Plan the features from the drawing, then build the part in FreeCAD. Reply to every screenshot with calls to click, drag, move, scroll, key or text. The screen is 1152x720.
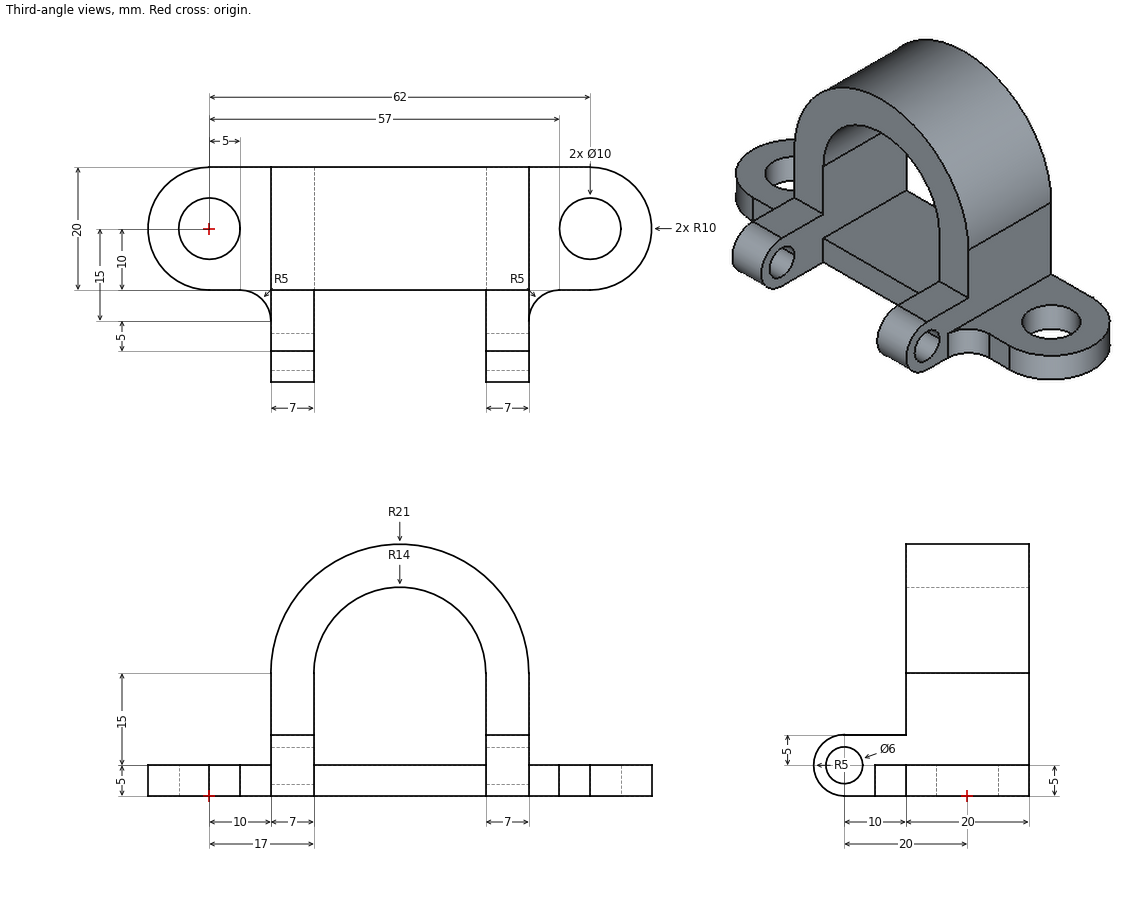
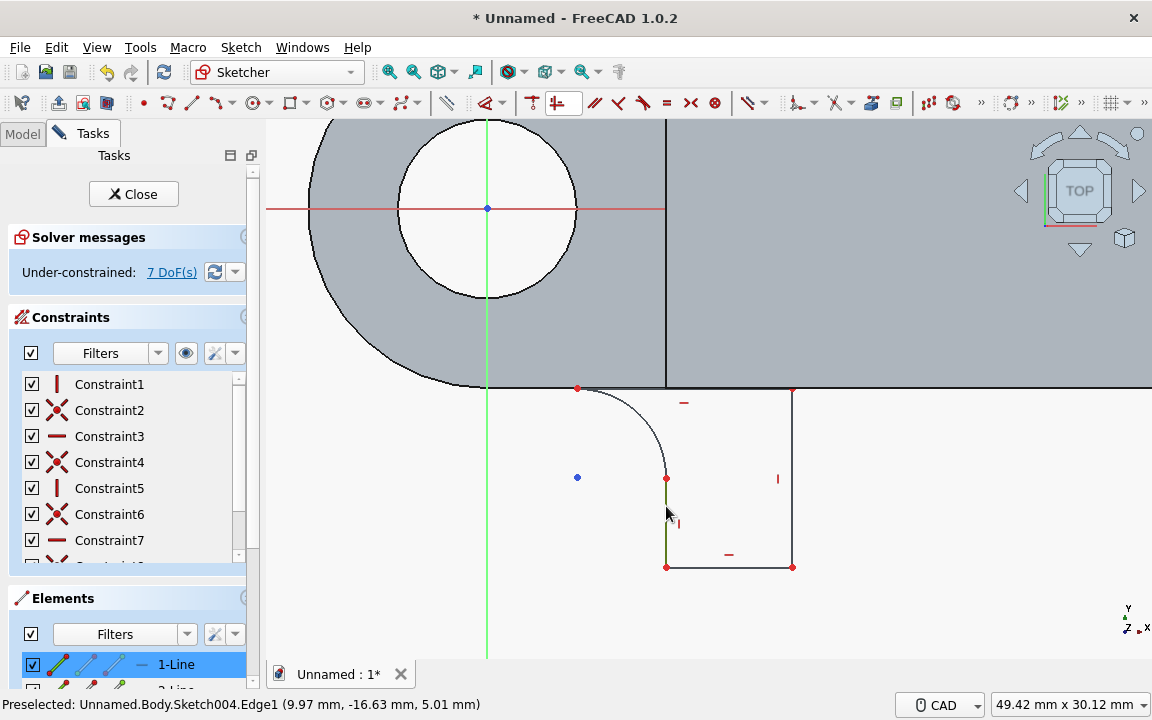
click(657, 438)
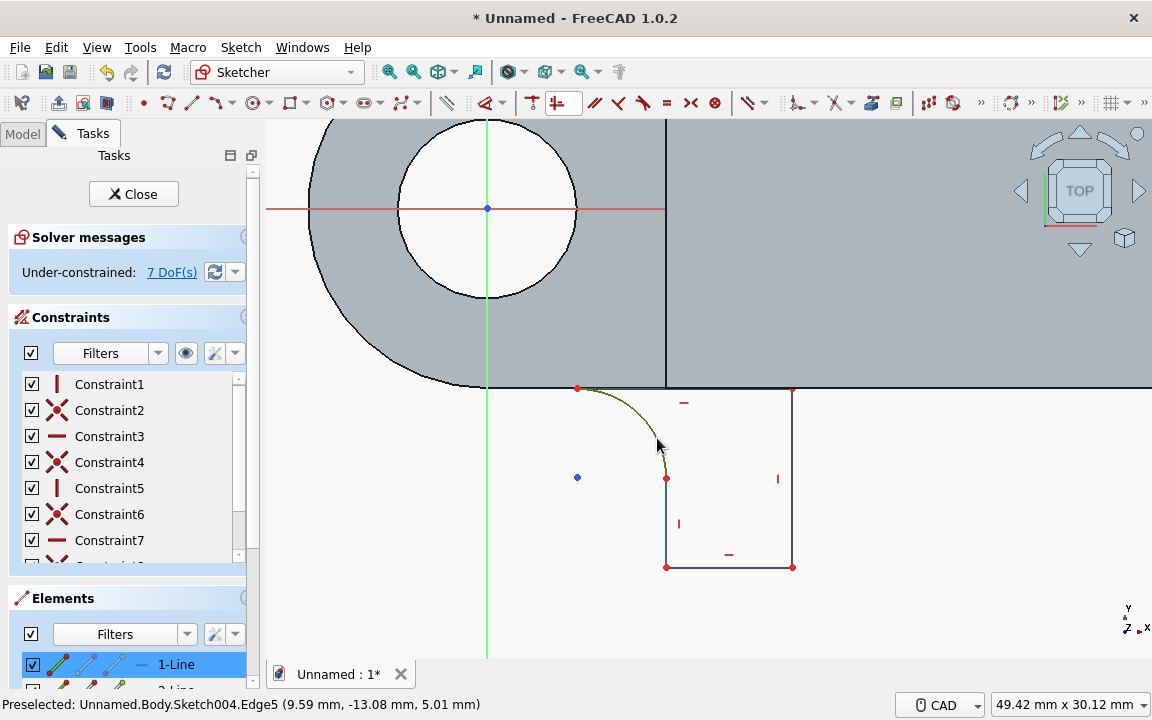
click(644, 104)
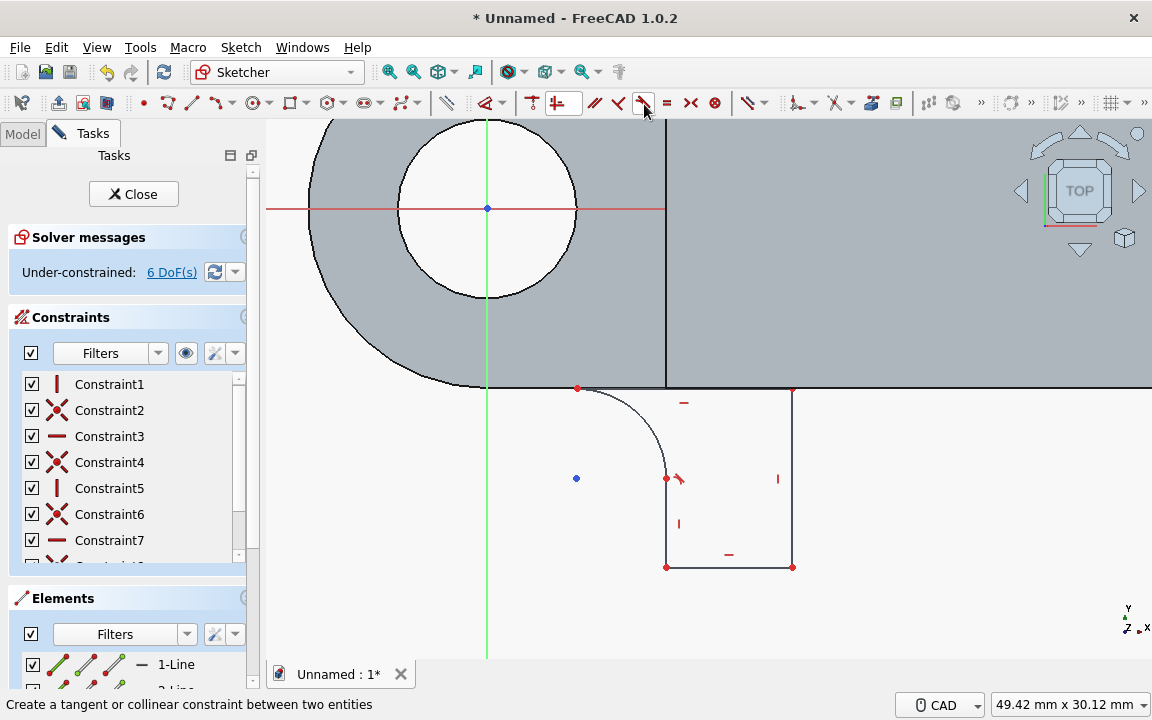
click(728, 389)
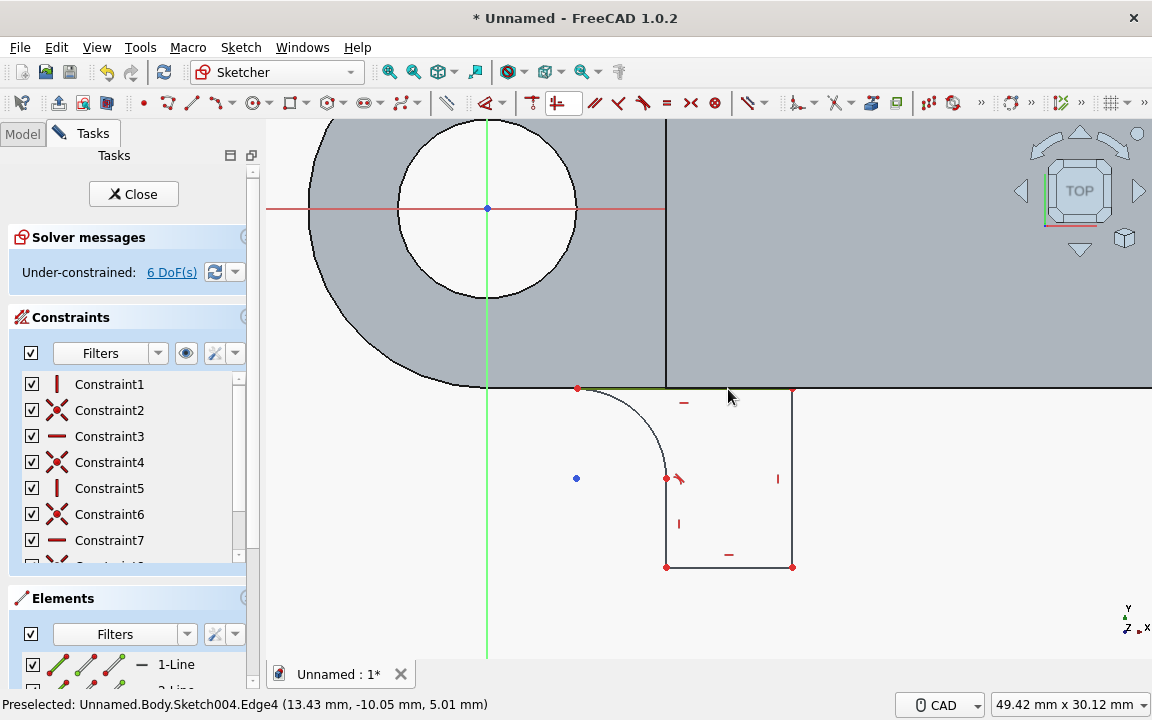
click(656, 438)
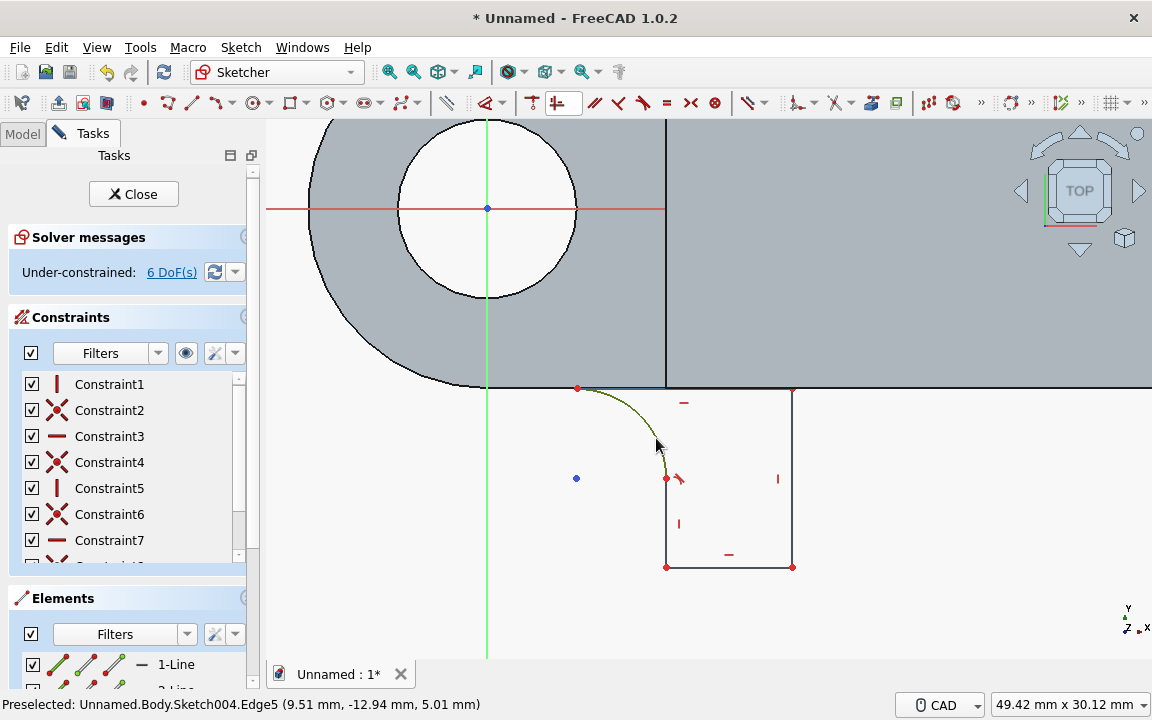
click(644, 104)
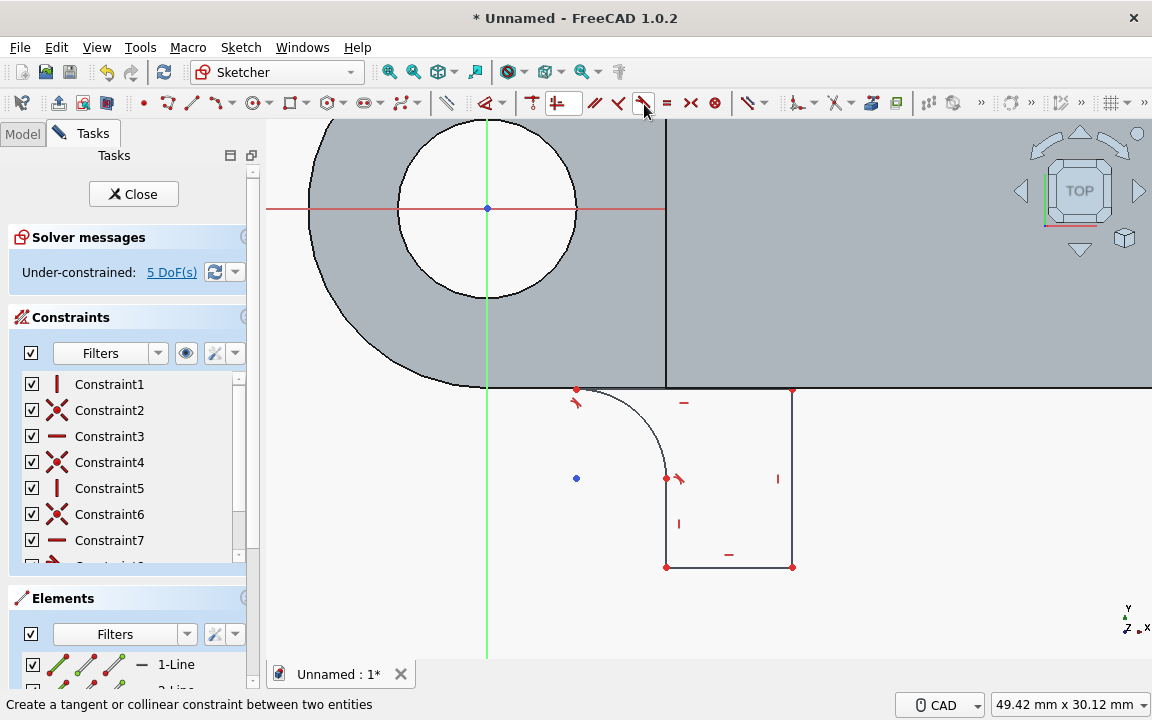
key(d)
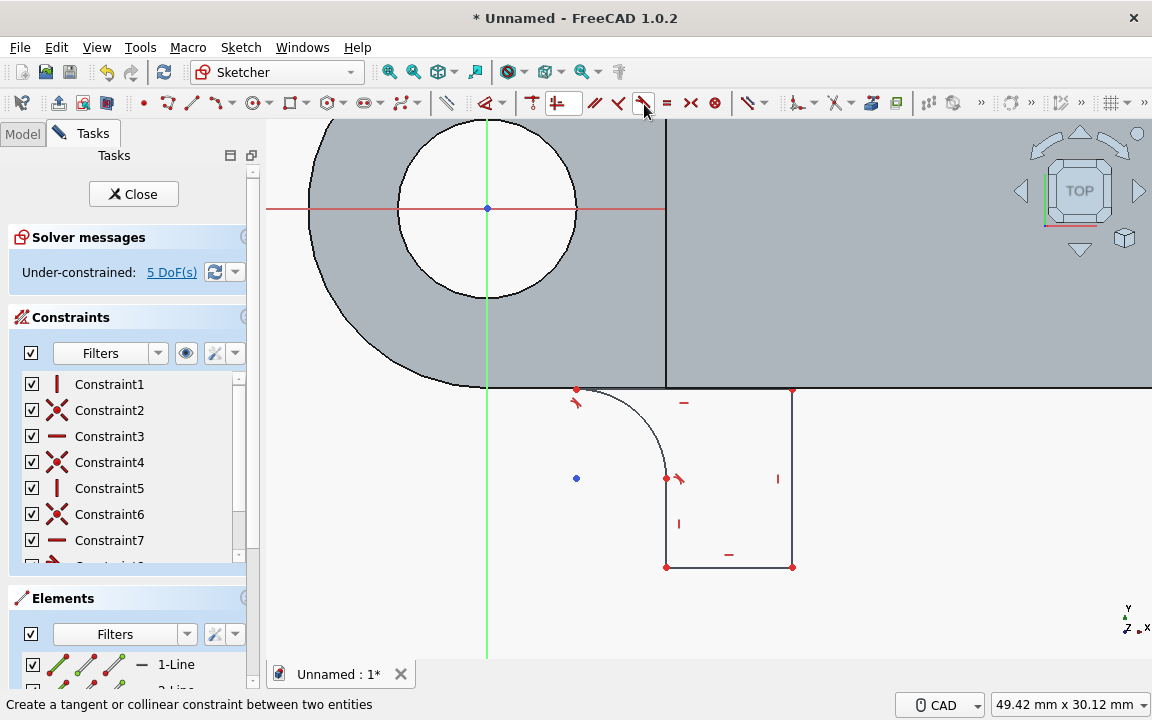
click(656, 438)
click(684, 423)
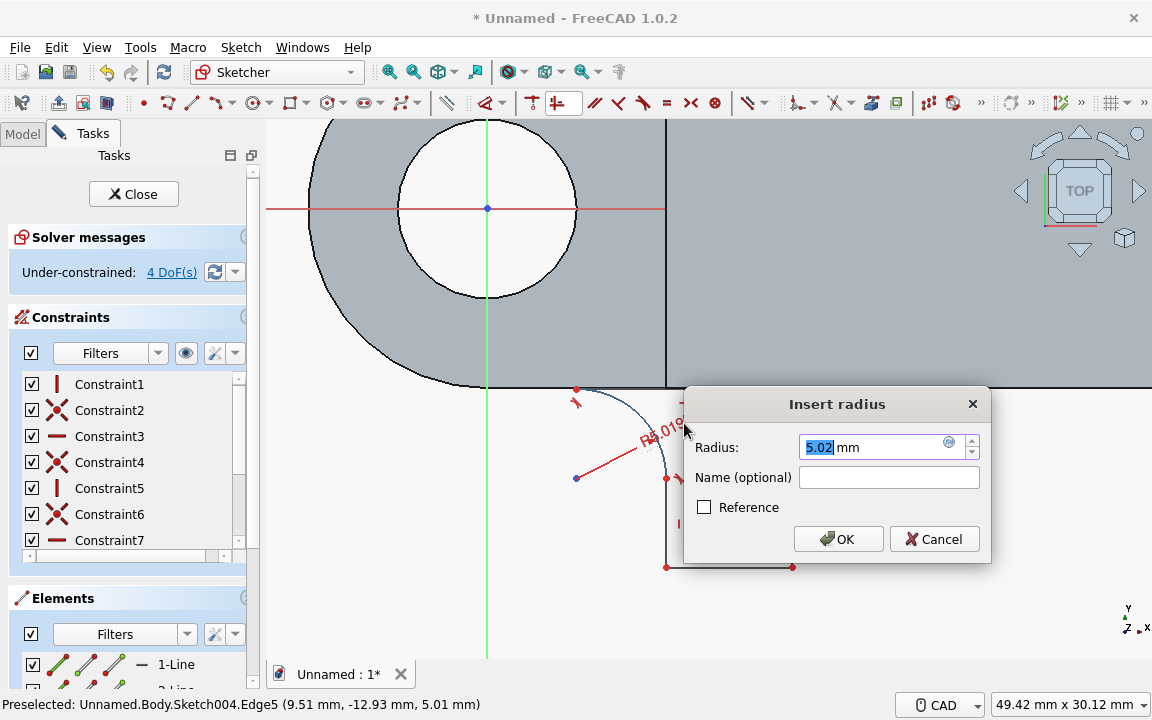
text(5)
key(Return)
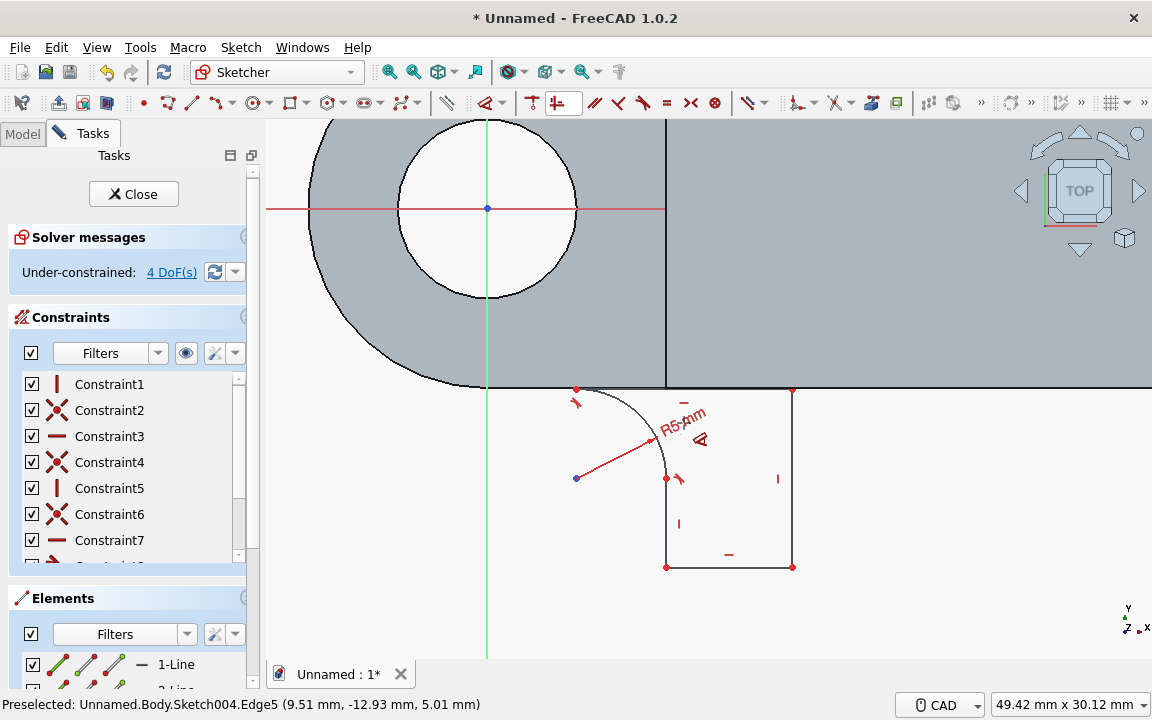
click(666, 505)
click(700, 523)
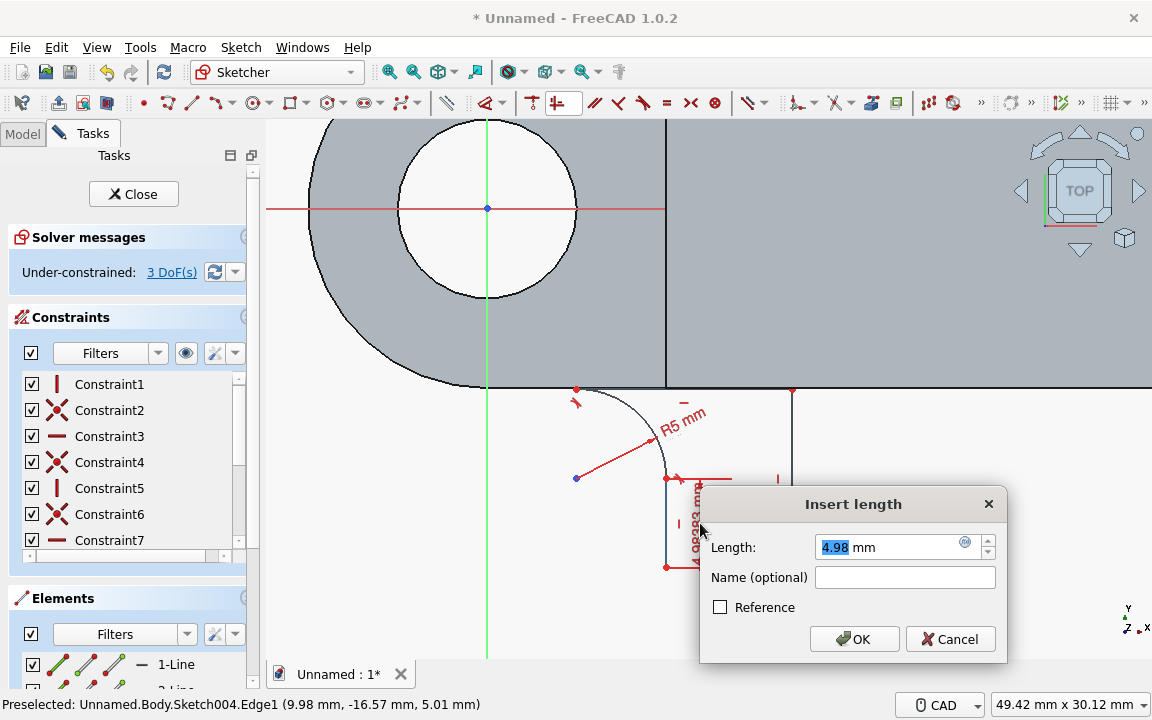
text(5)
key(Return)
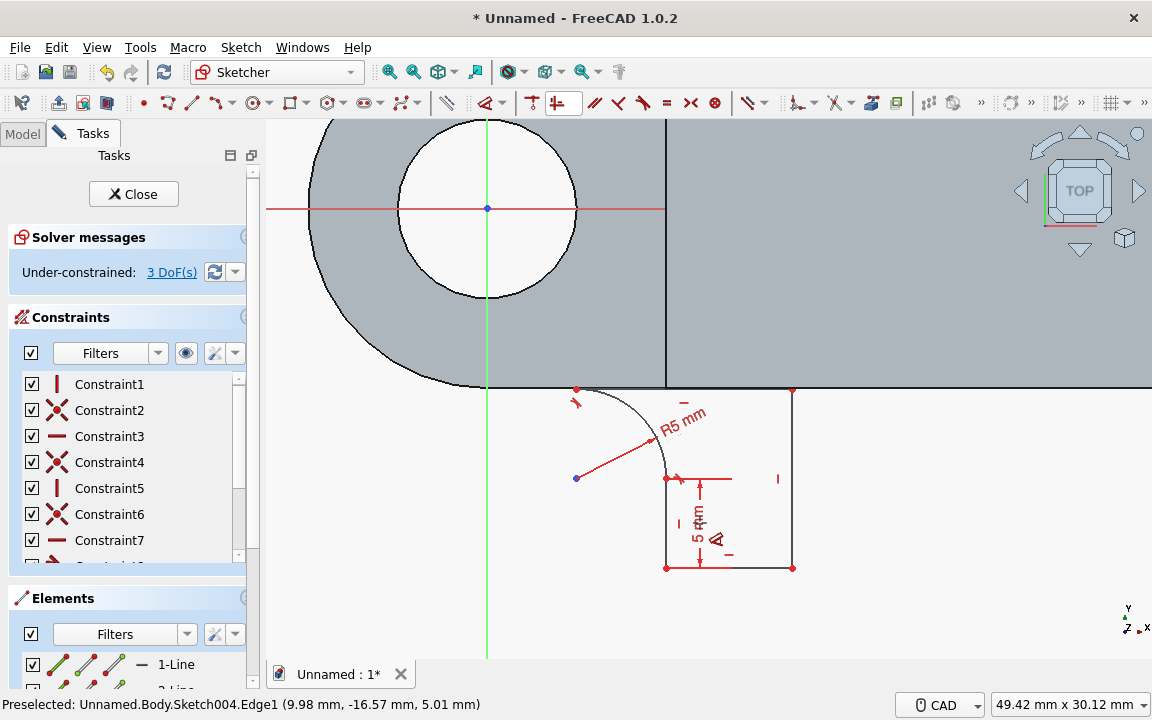
click(704, 568)
click(729, 602)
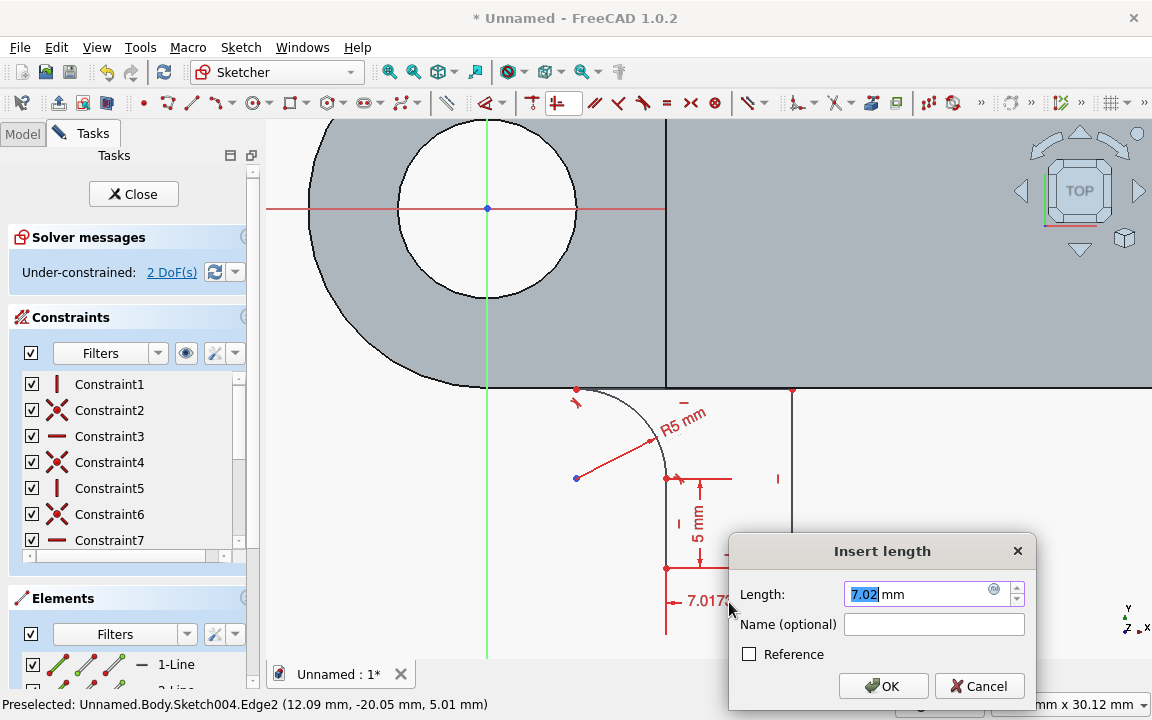
text(7)
key(Return)